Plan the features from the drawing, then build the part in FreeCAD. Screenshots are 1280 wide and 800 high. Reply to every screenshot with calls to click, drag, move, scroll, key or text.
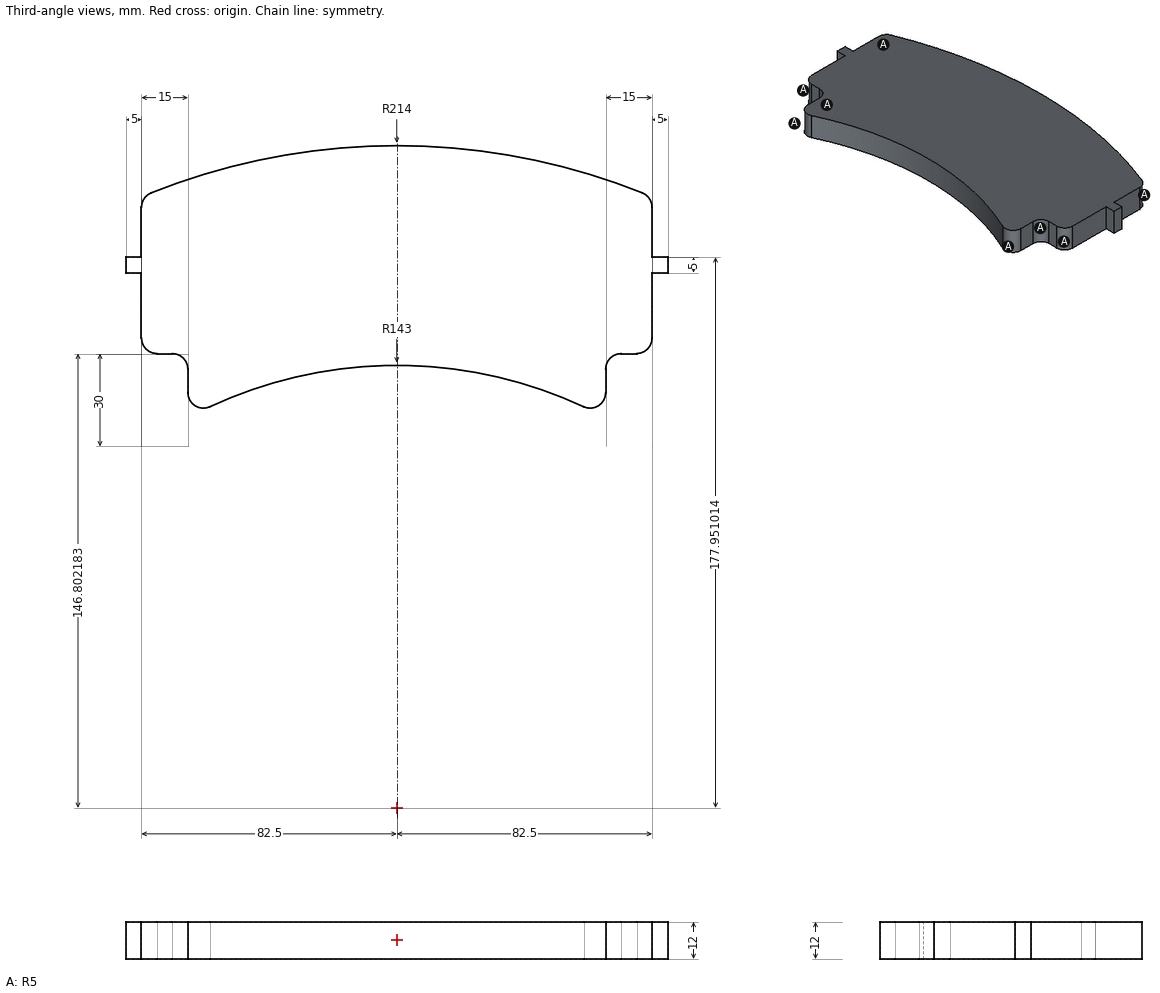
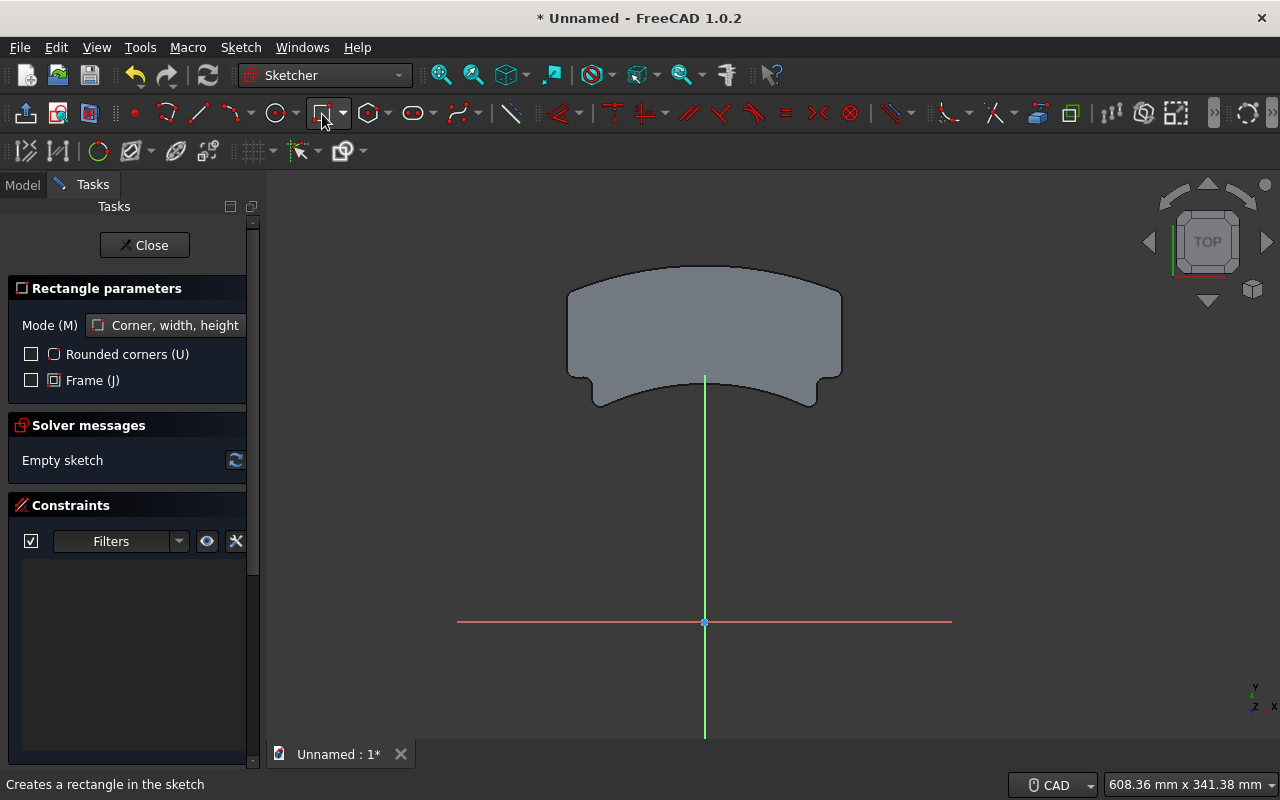
scroll(842, 326, up, 4)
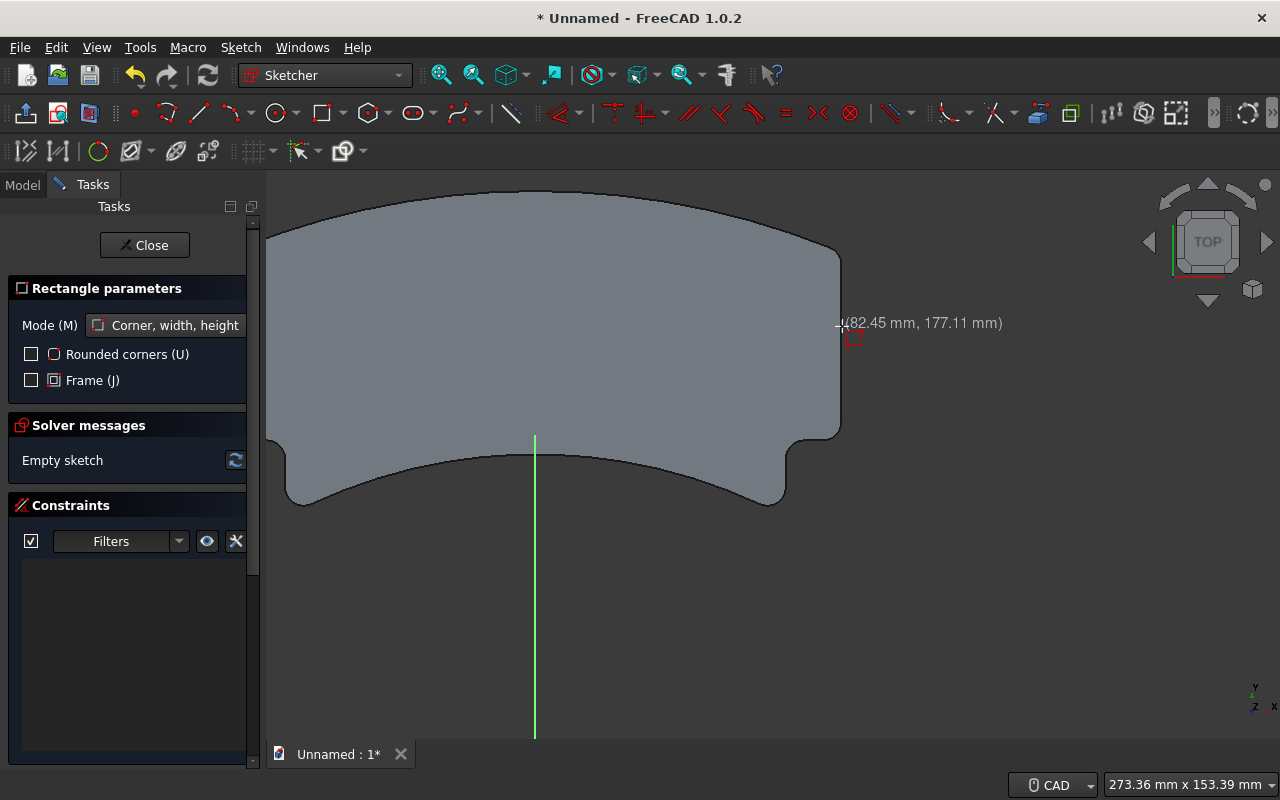
click(841, 325)
move(860, 343)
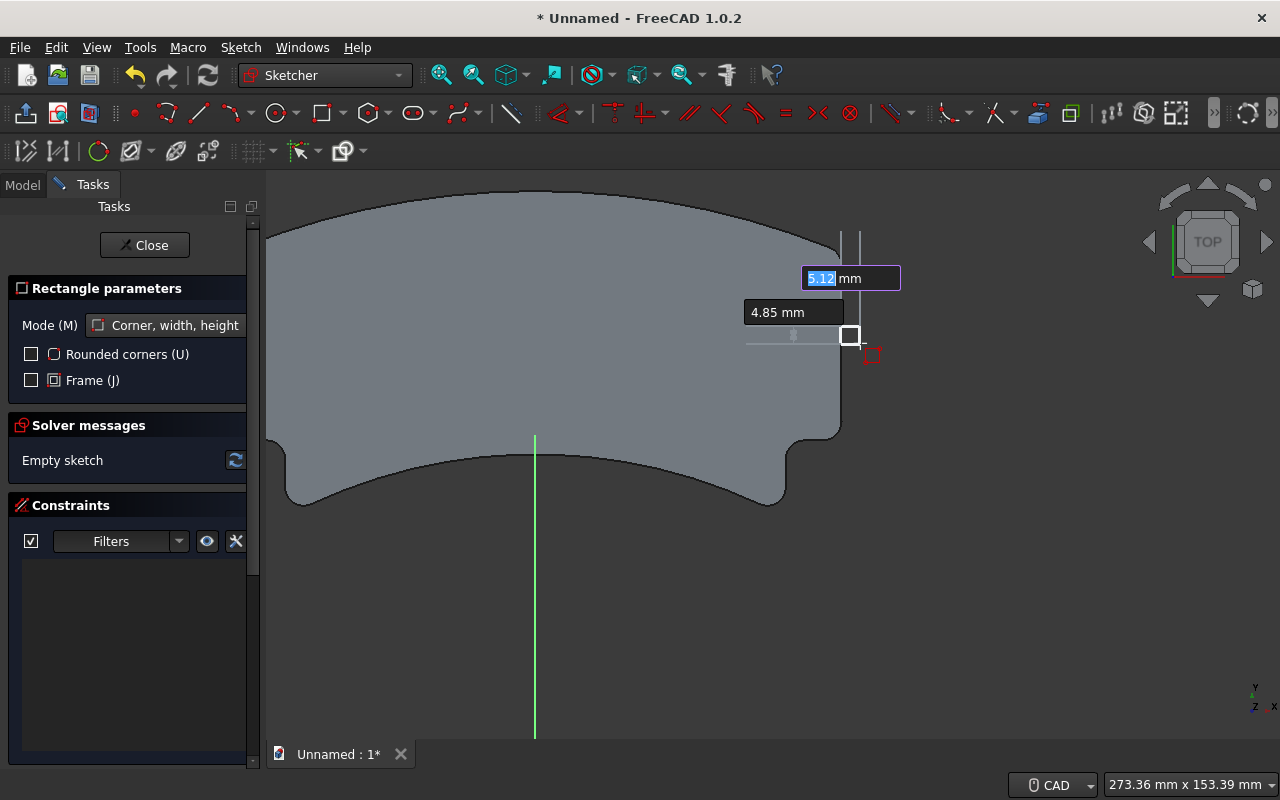
text(5)
key(Tab)
text(5)
key(Return)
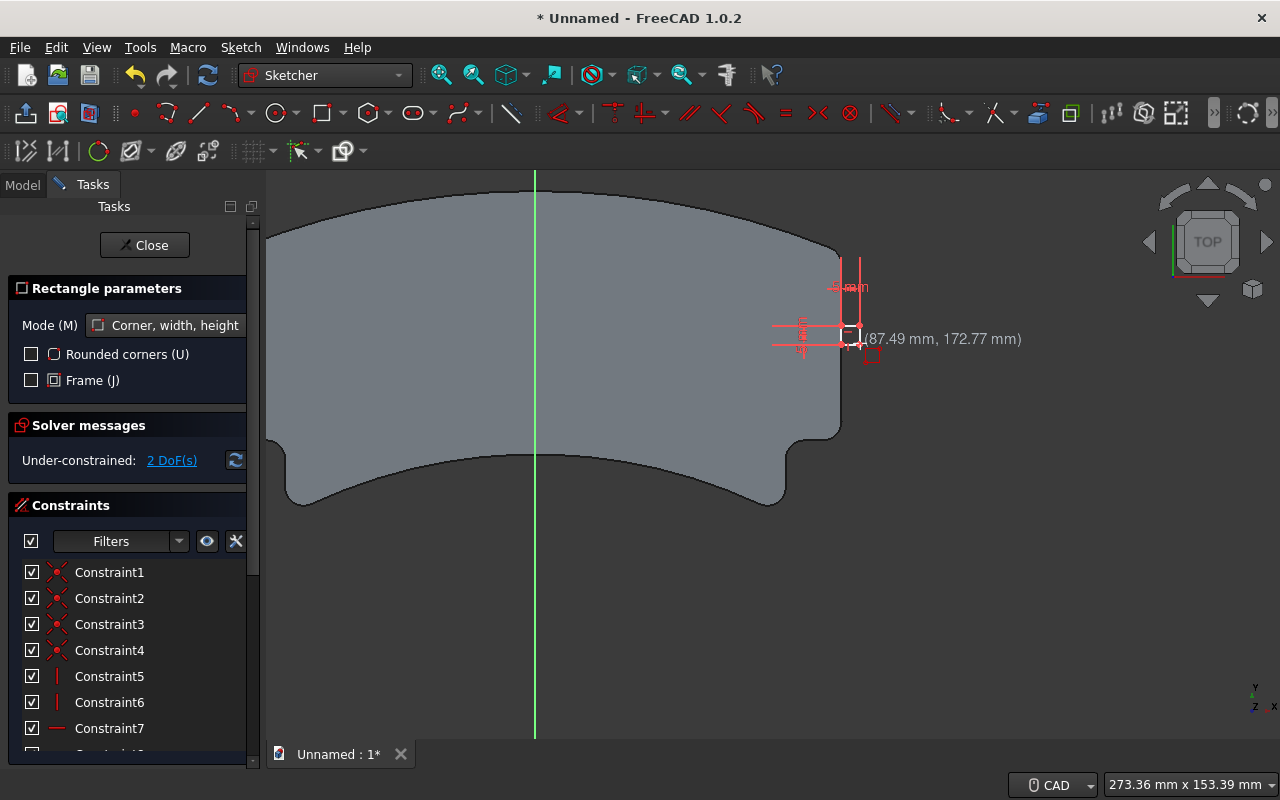
scroll(910, 211, down, 3)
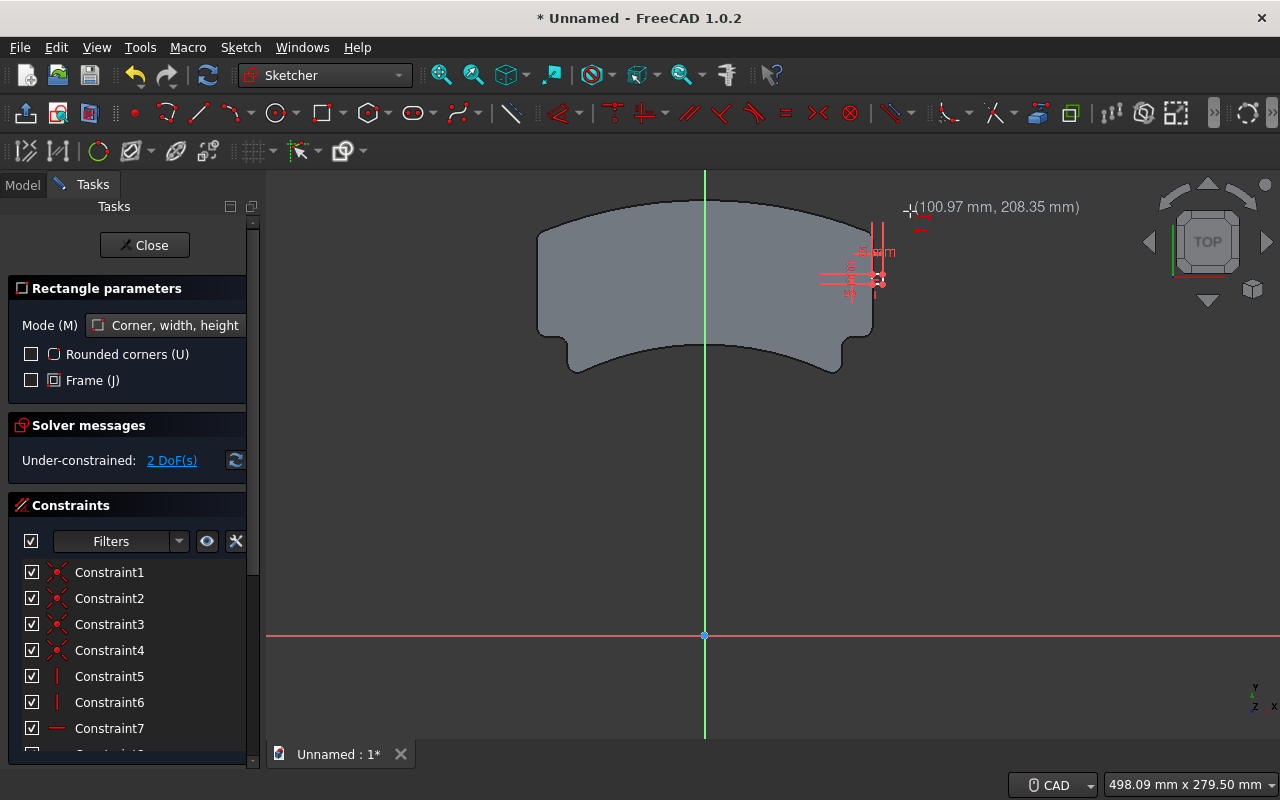
scroll(527, 273, up, 3)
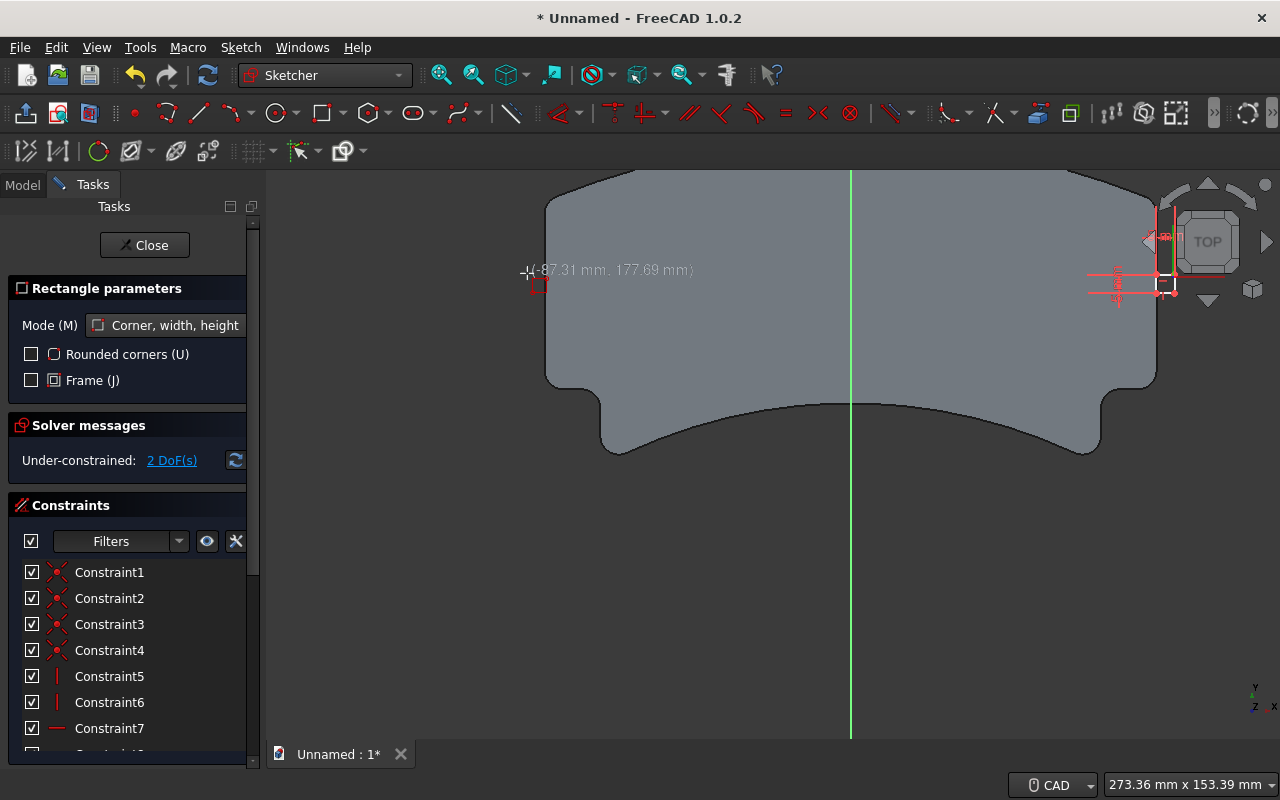
click(526, 274)
move(545, 292)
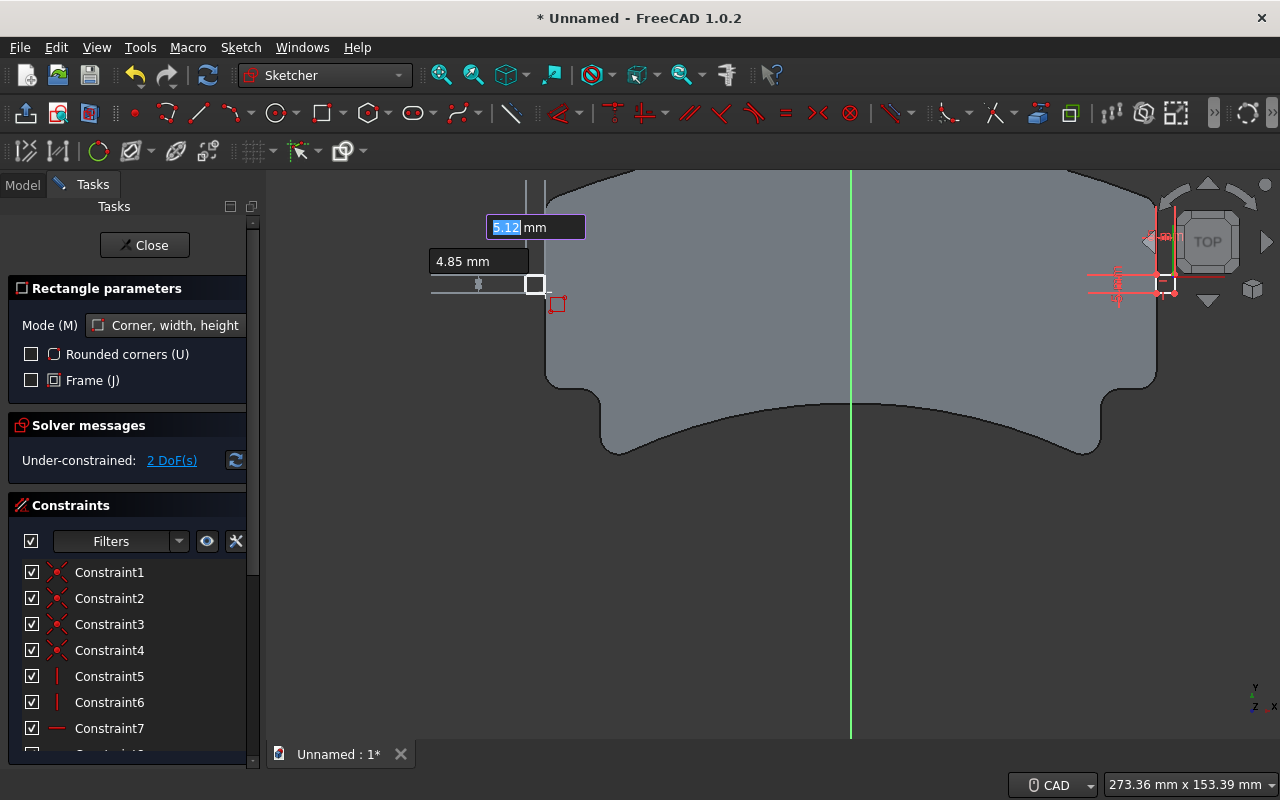
text(5)
key(Tab)
text(5)
key(Return)
key(Escape)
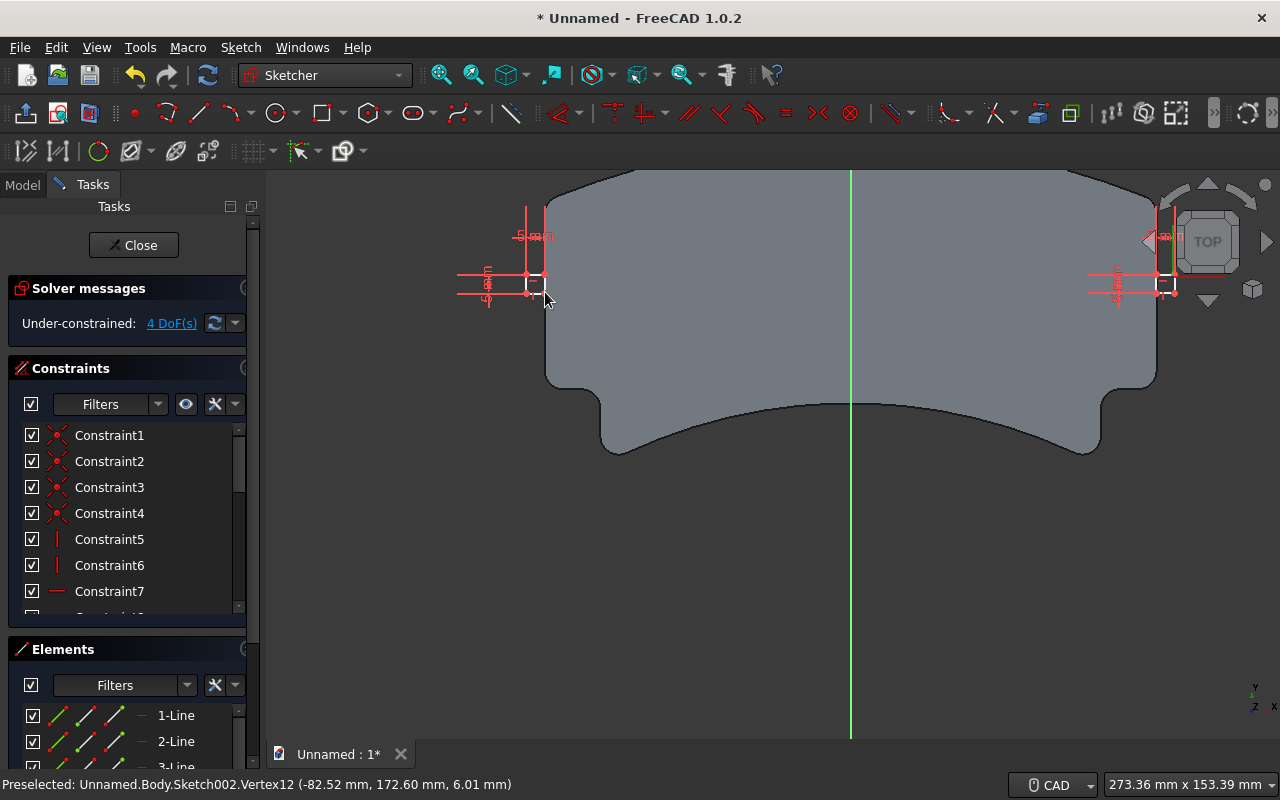
scroll(527, 273, down, 3)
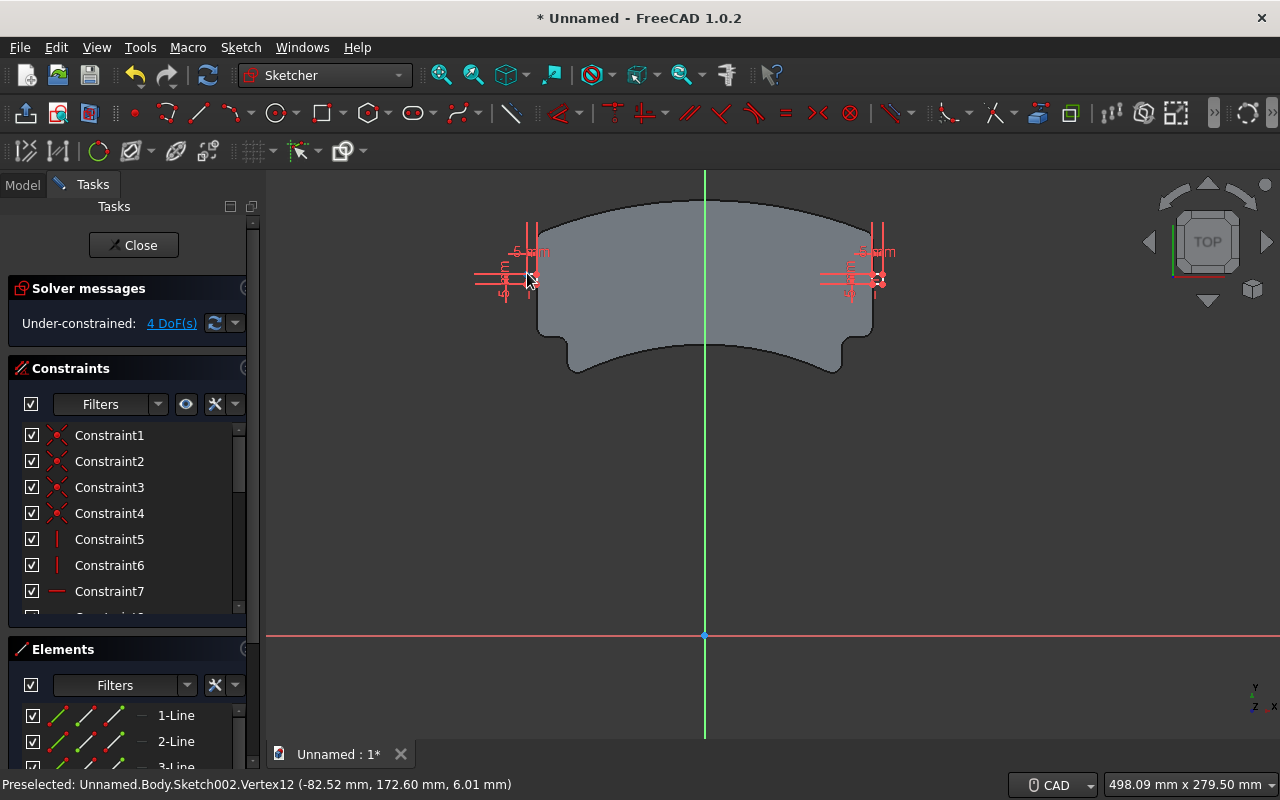
click(883, 274)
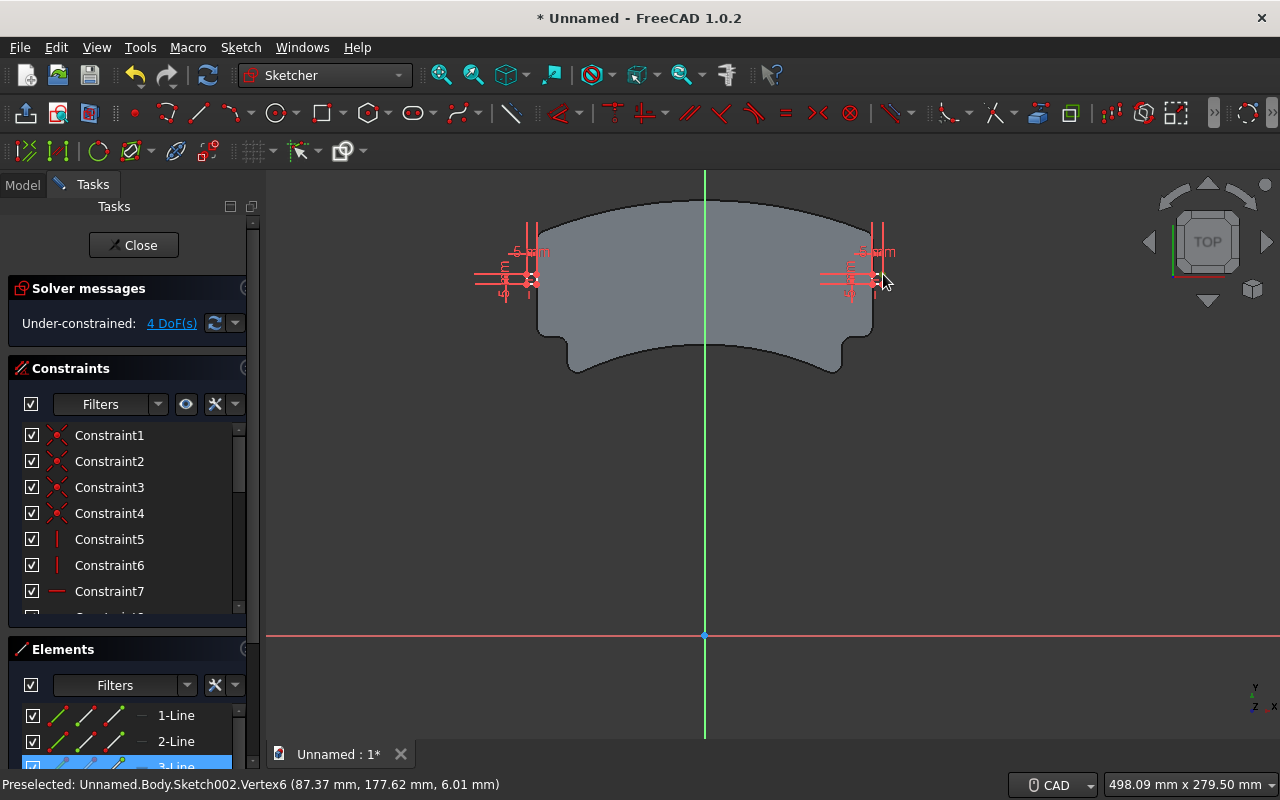
click(527, 274)